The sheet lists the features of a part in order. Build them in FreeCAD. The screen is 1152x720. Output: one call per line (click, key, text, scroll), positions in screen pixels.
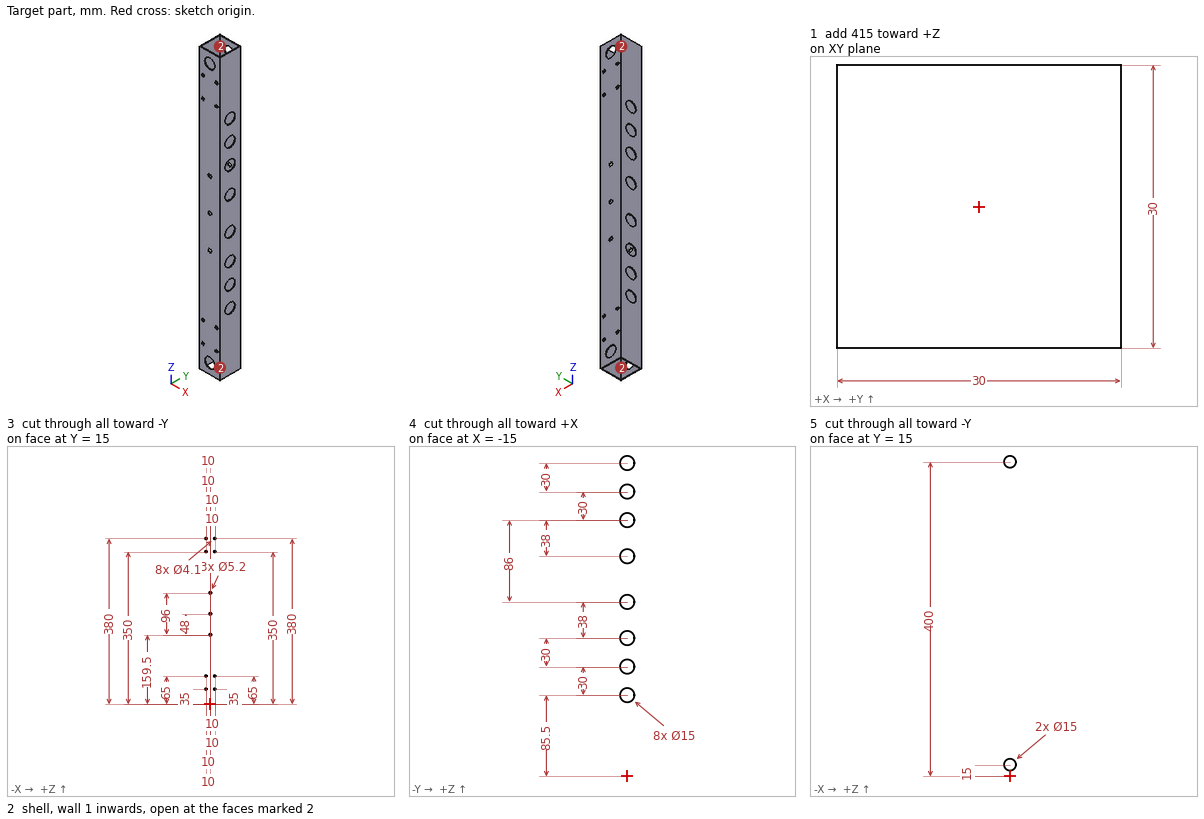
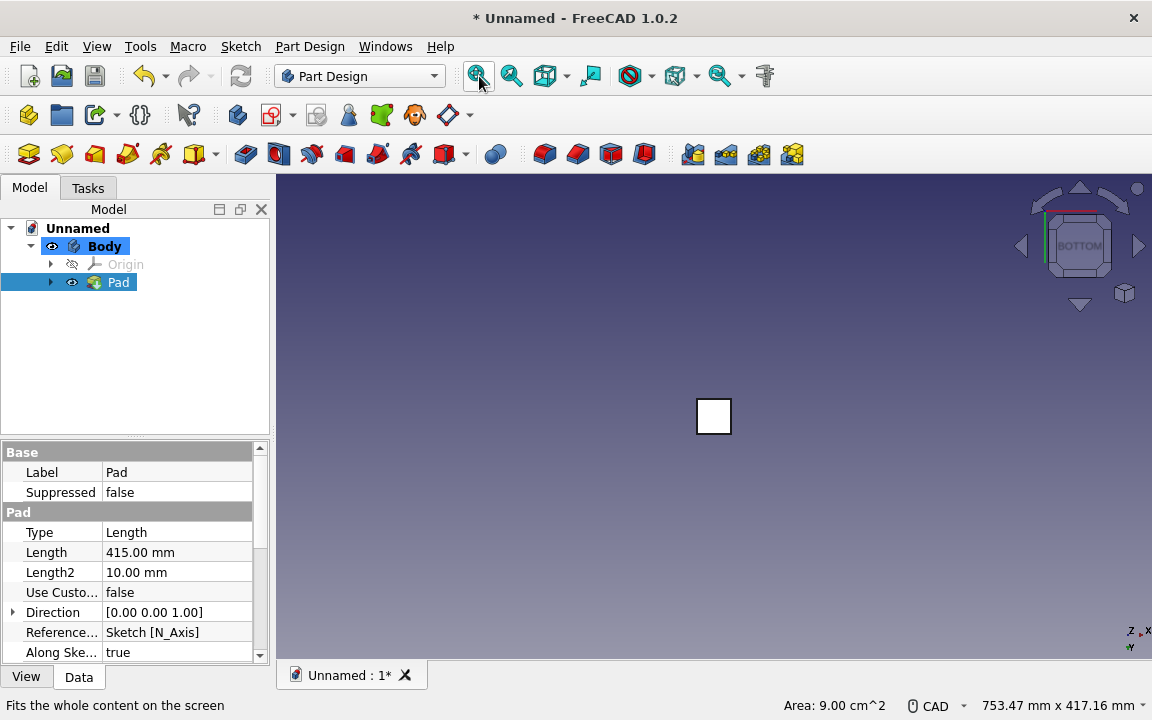
key(v)
key(f)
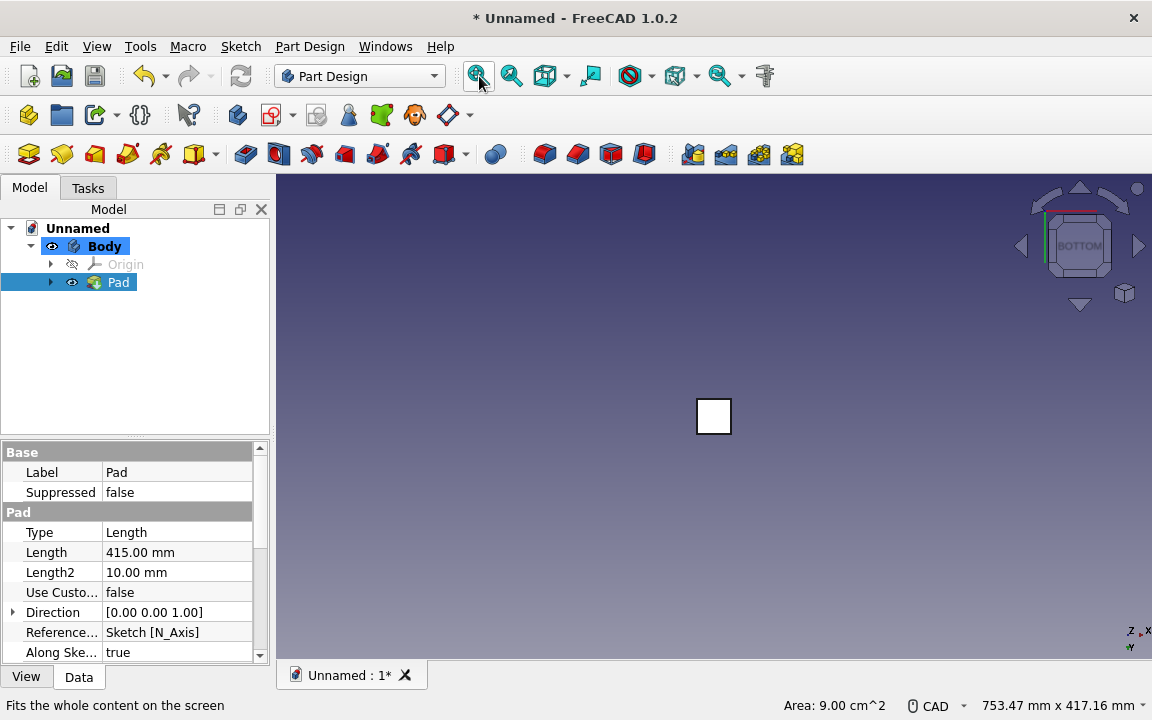
click(714, 415, ctrl)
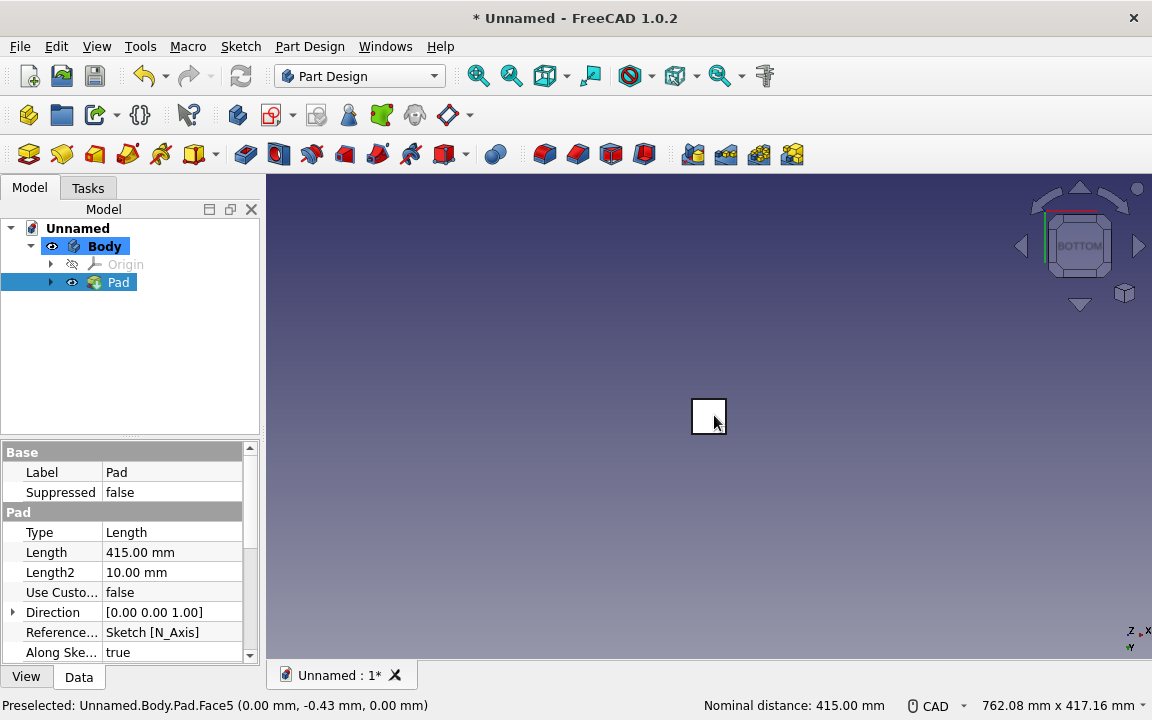
click(644, 154)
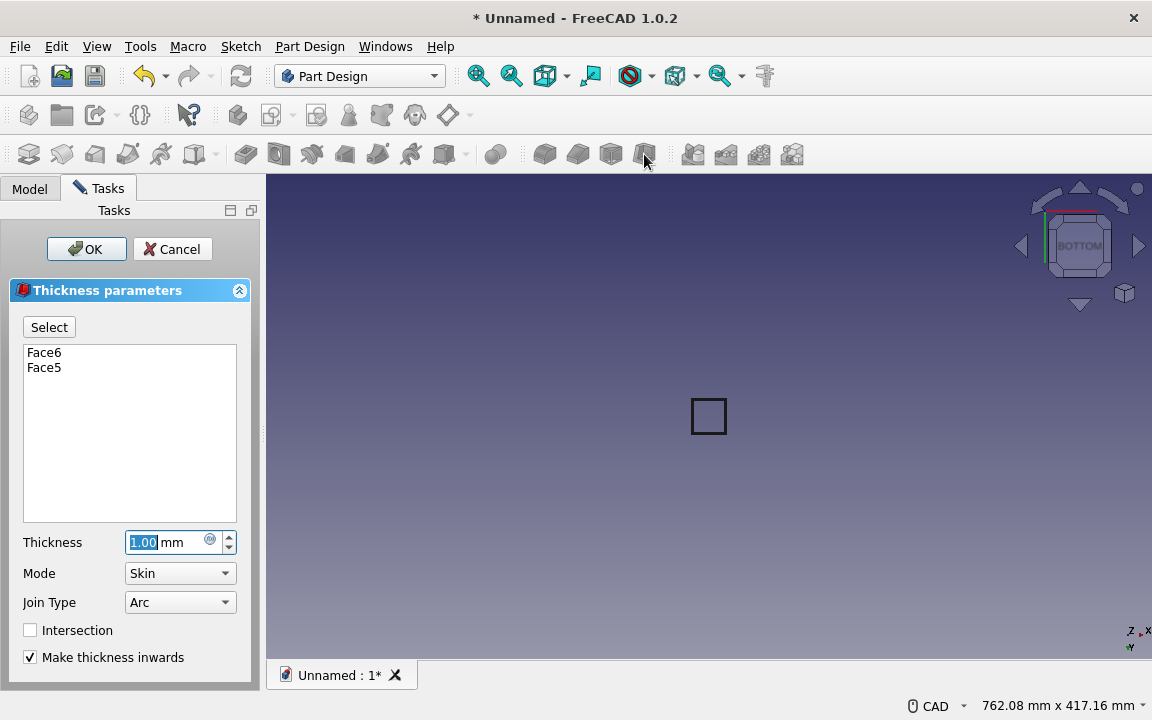
text(1)
key(Tab)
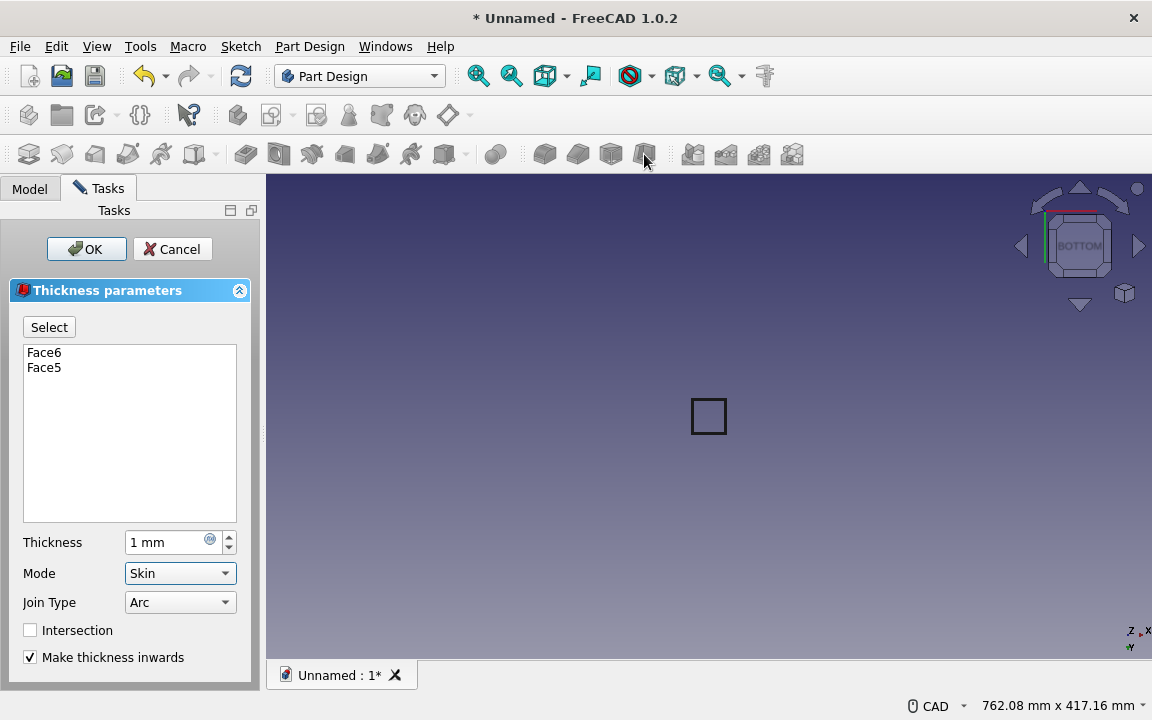
click(181, 602)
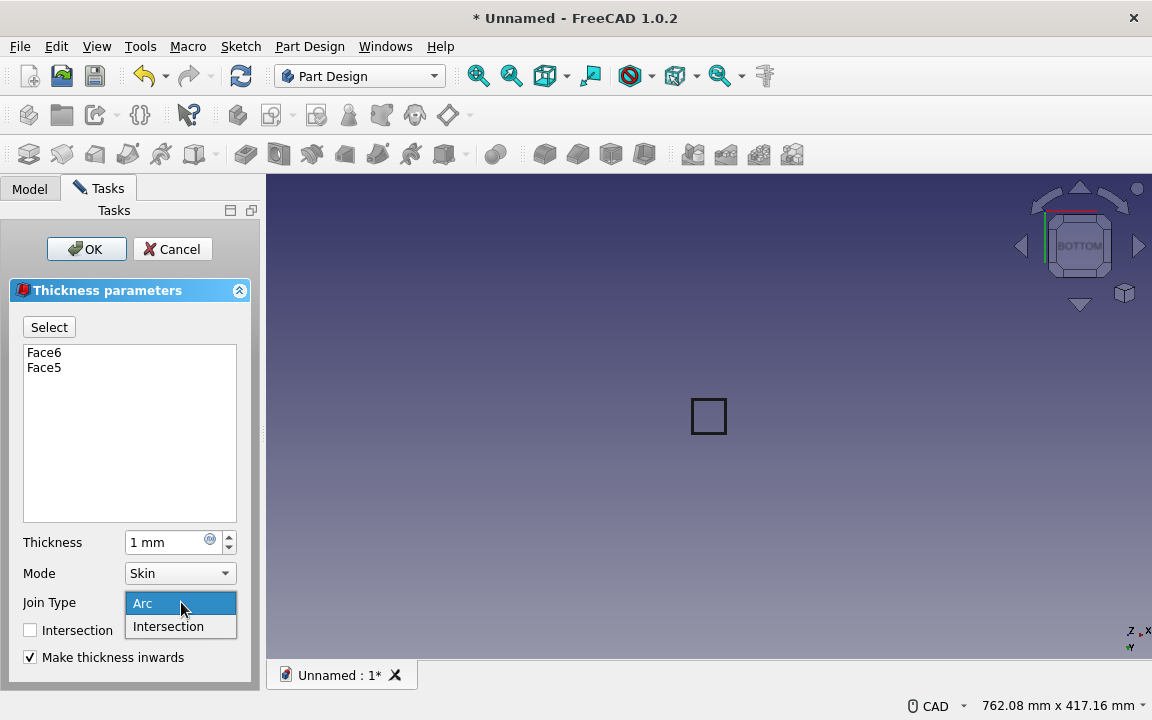
click(179, 626)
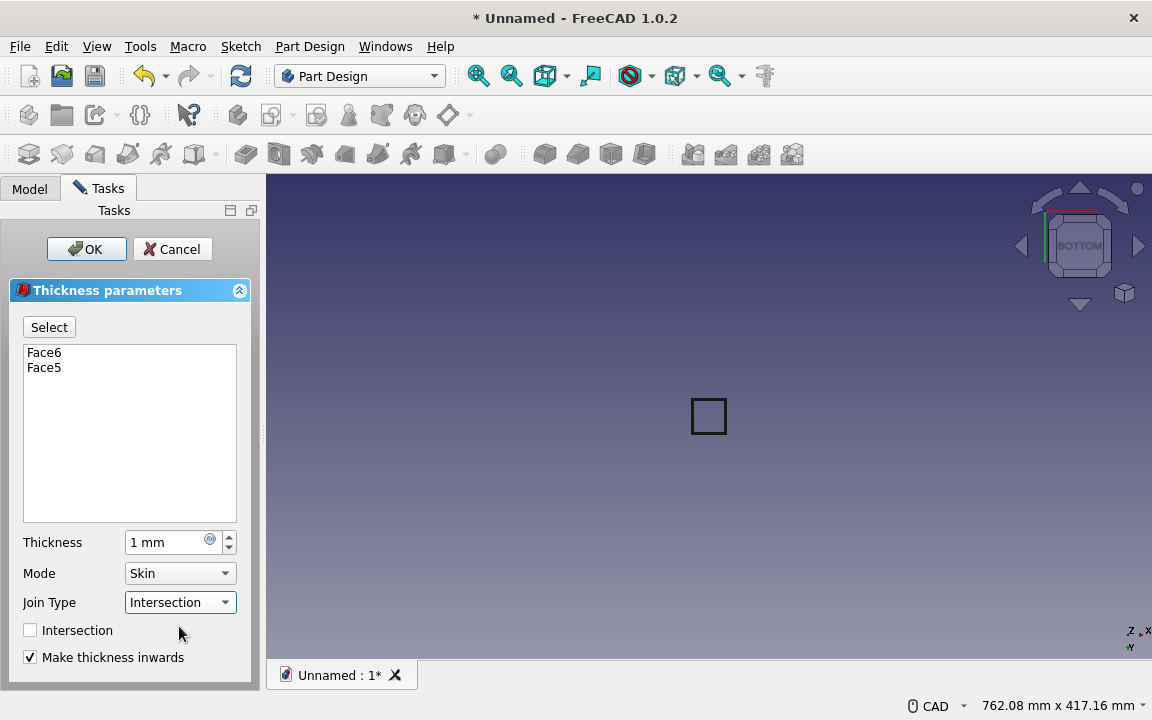
click(87, 249)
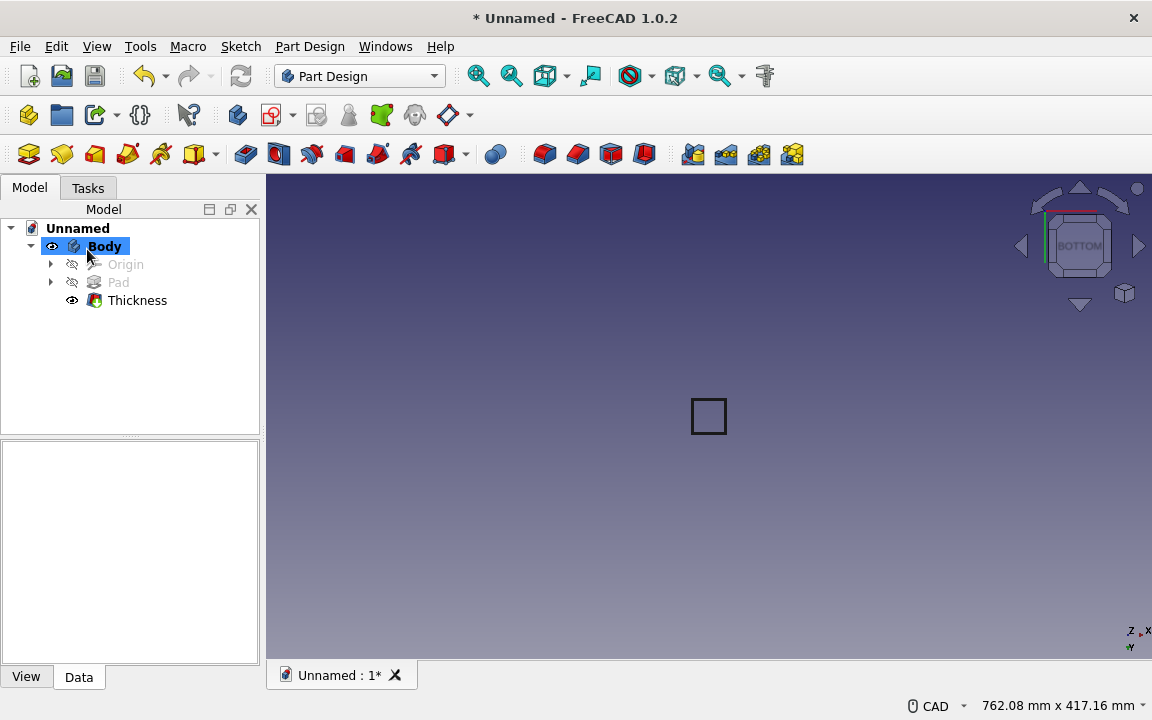
key(v)
key(f)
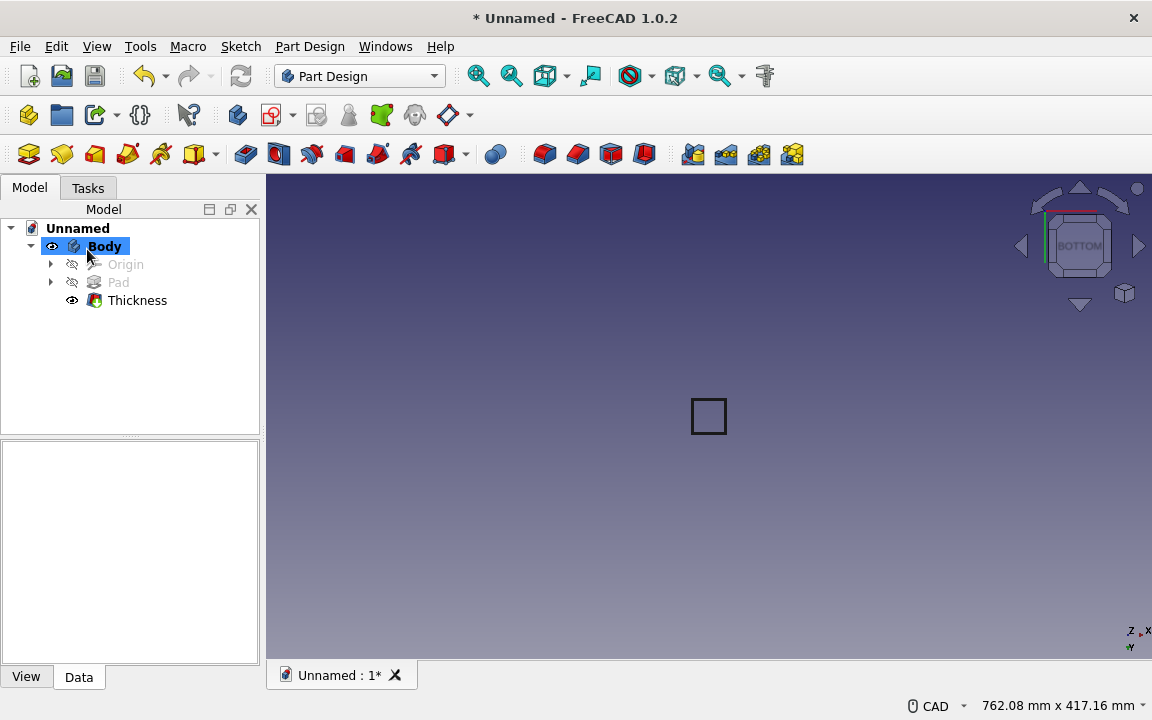
key(4)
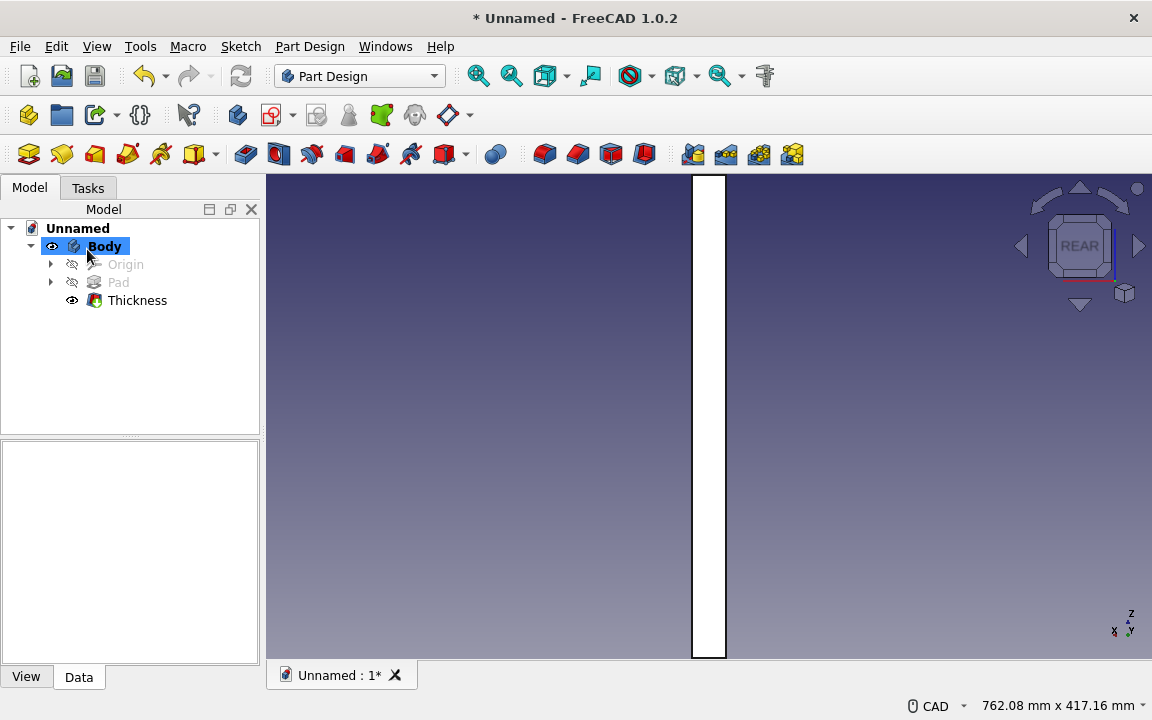
click(709, 209)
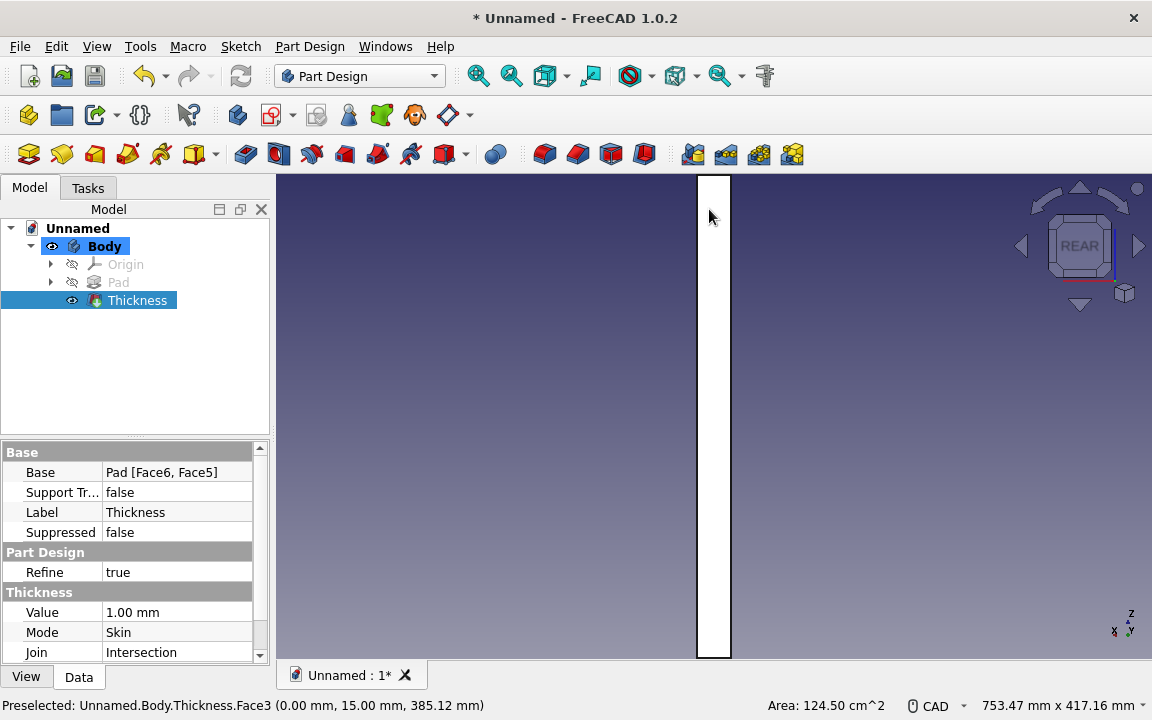
click(270, 116)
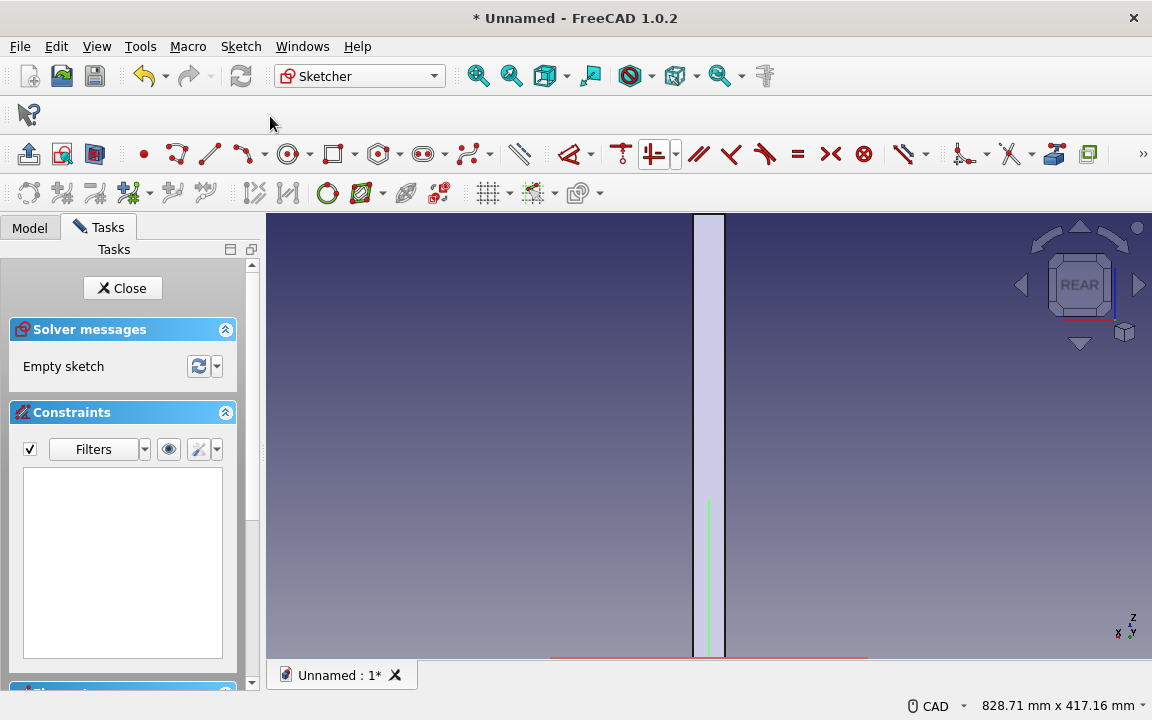
scroll(501, 400, down, 2)